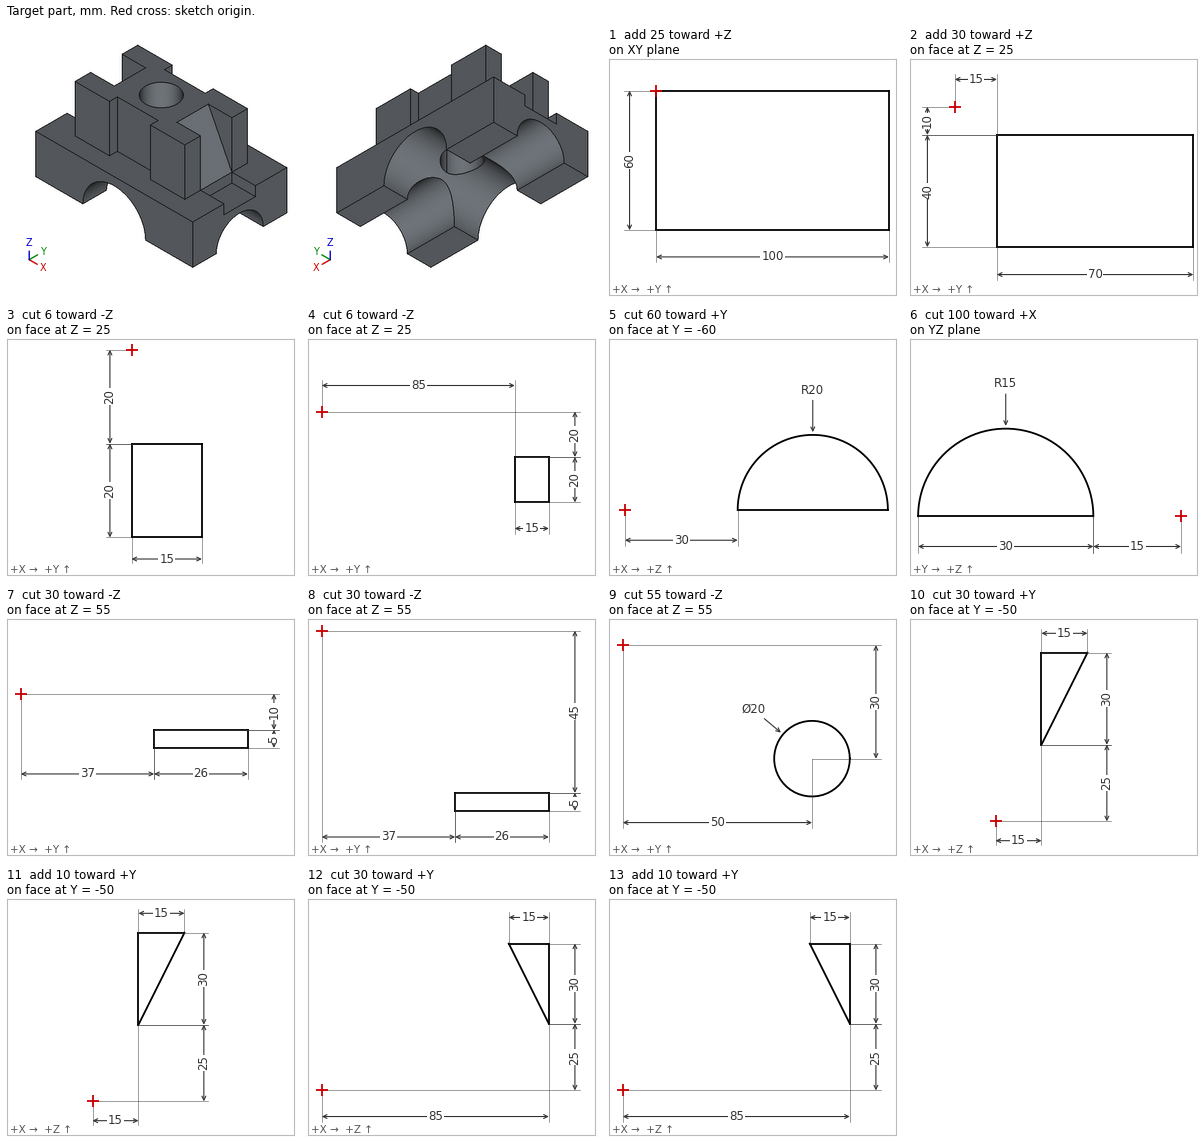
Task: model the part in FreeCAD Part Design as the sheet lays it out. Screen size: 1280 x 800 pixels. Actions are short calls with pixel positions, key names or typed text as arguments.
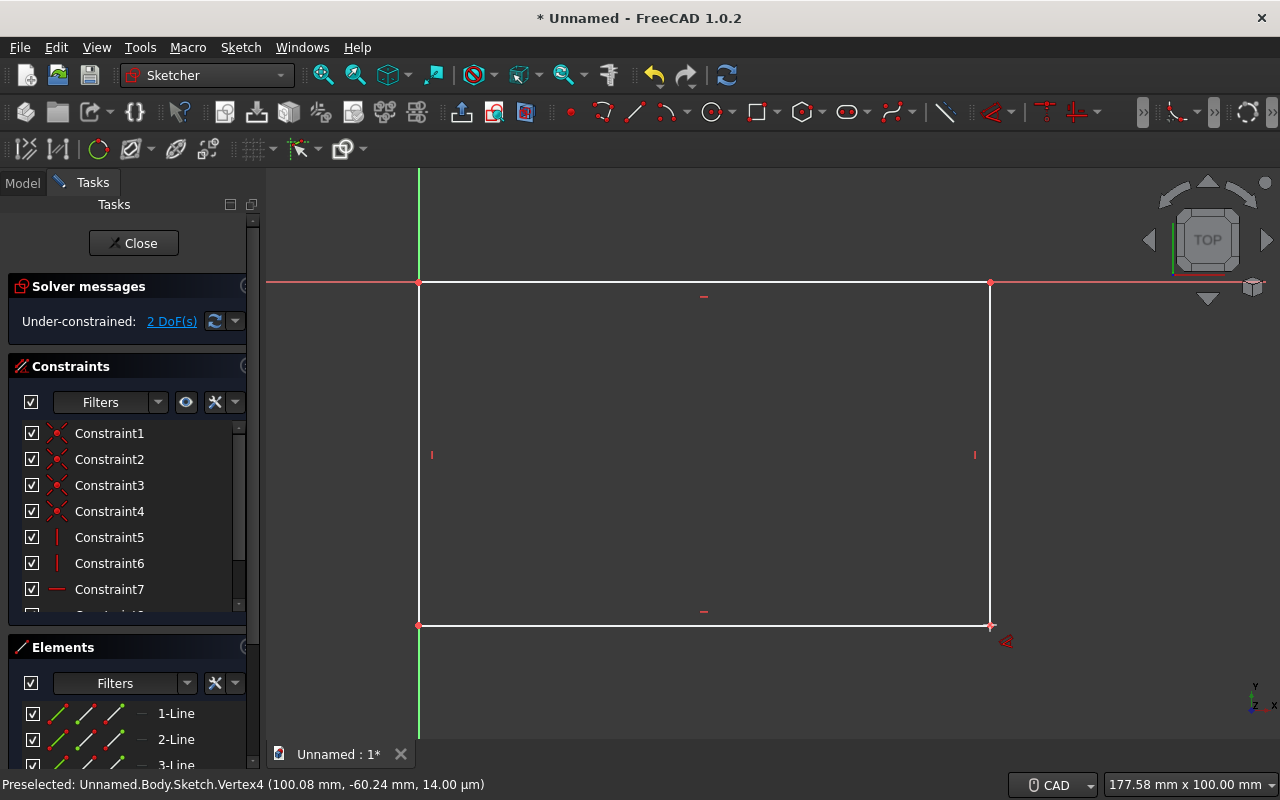
click(419, 385)
click(385, 454)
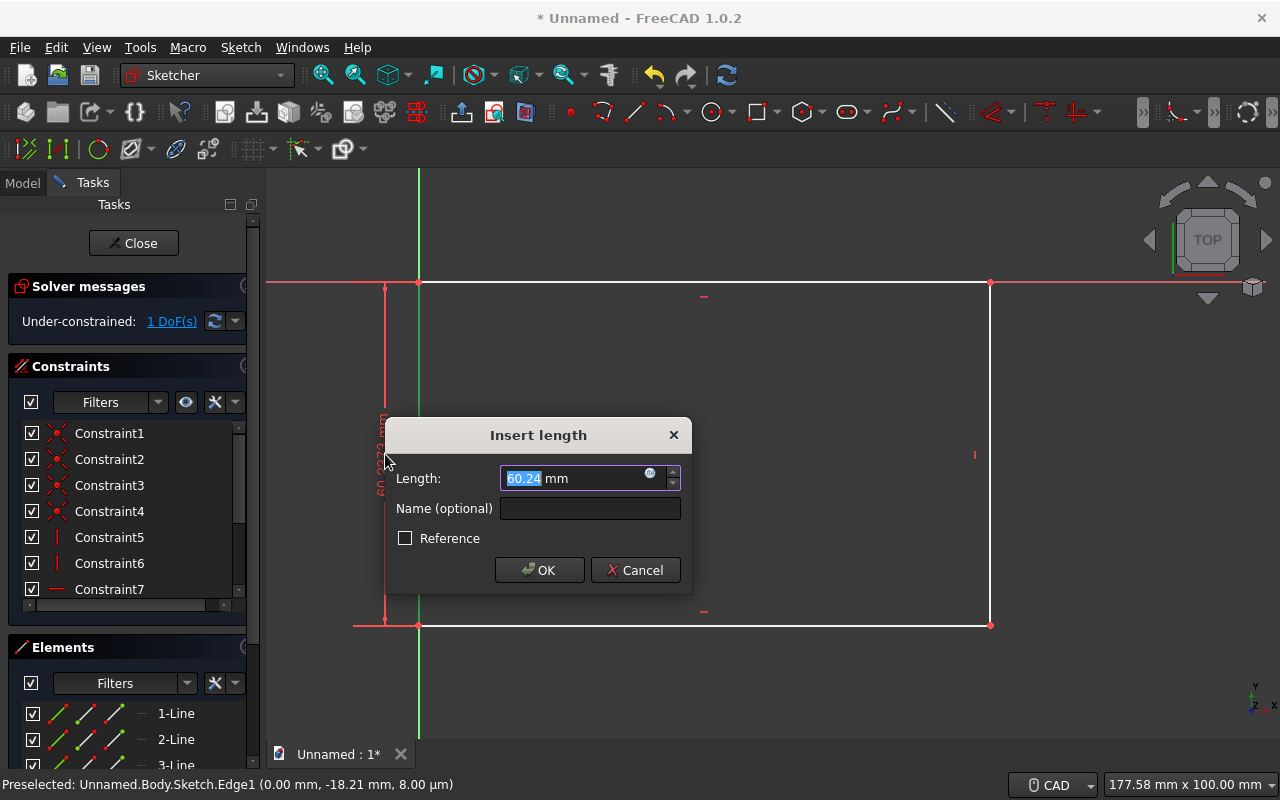
text(60)
key(Return)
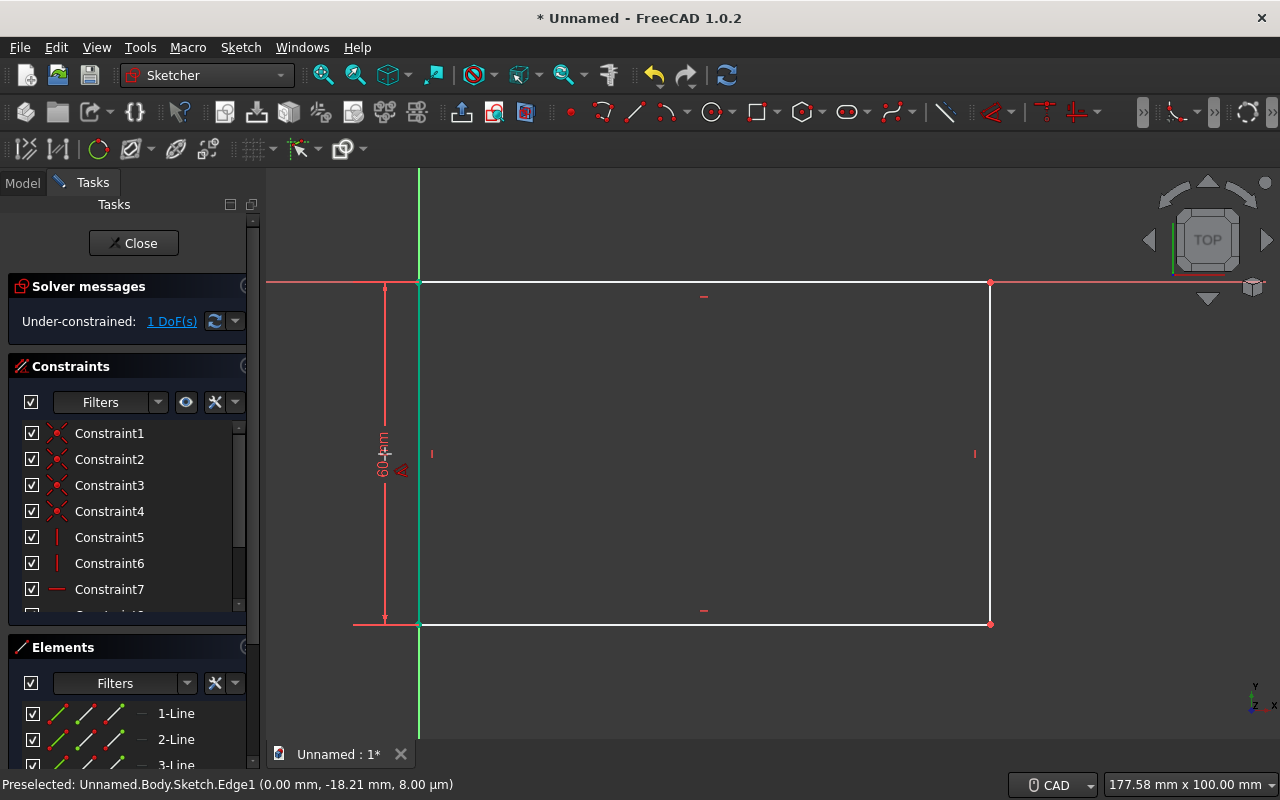
click(590, 625)
click(704, 659)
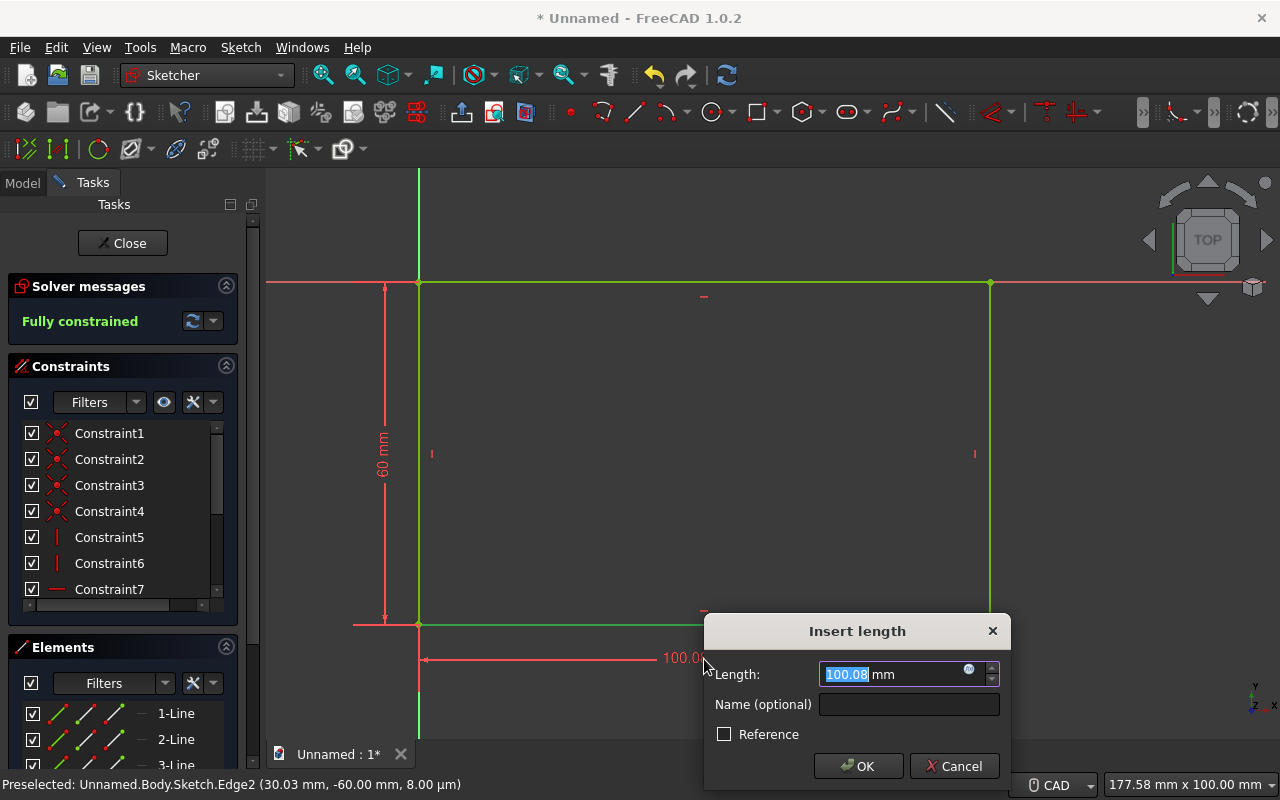
text(100)
key(Return)
key(Escape)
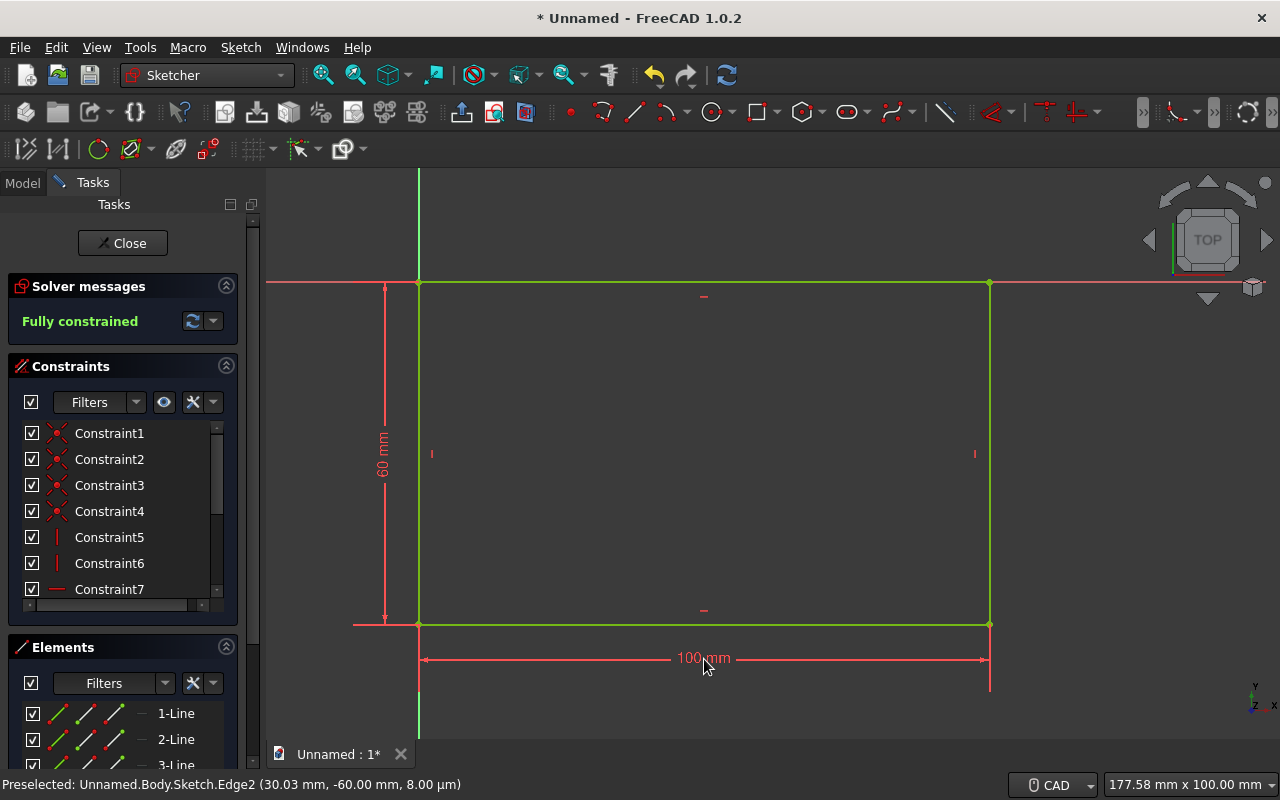
click(123, 243)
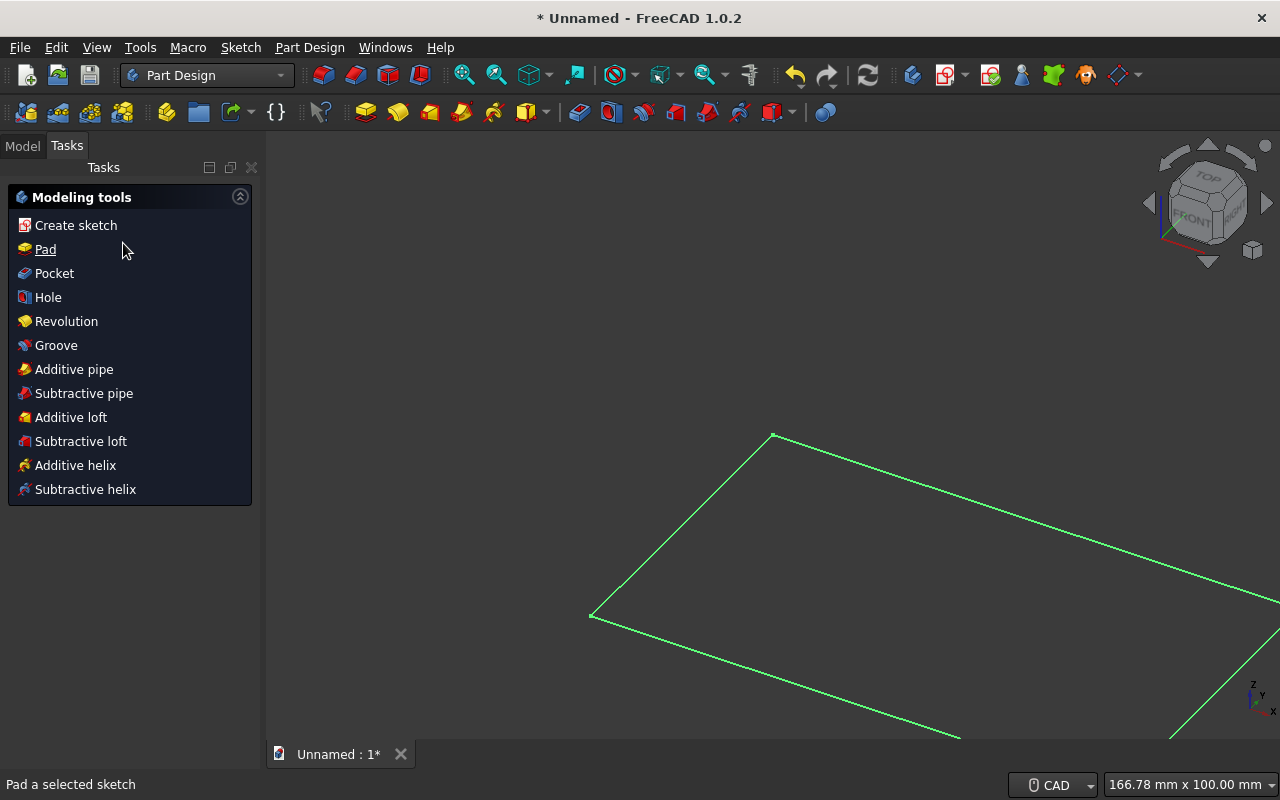
click(366, 112)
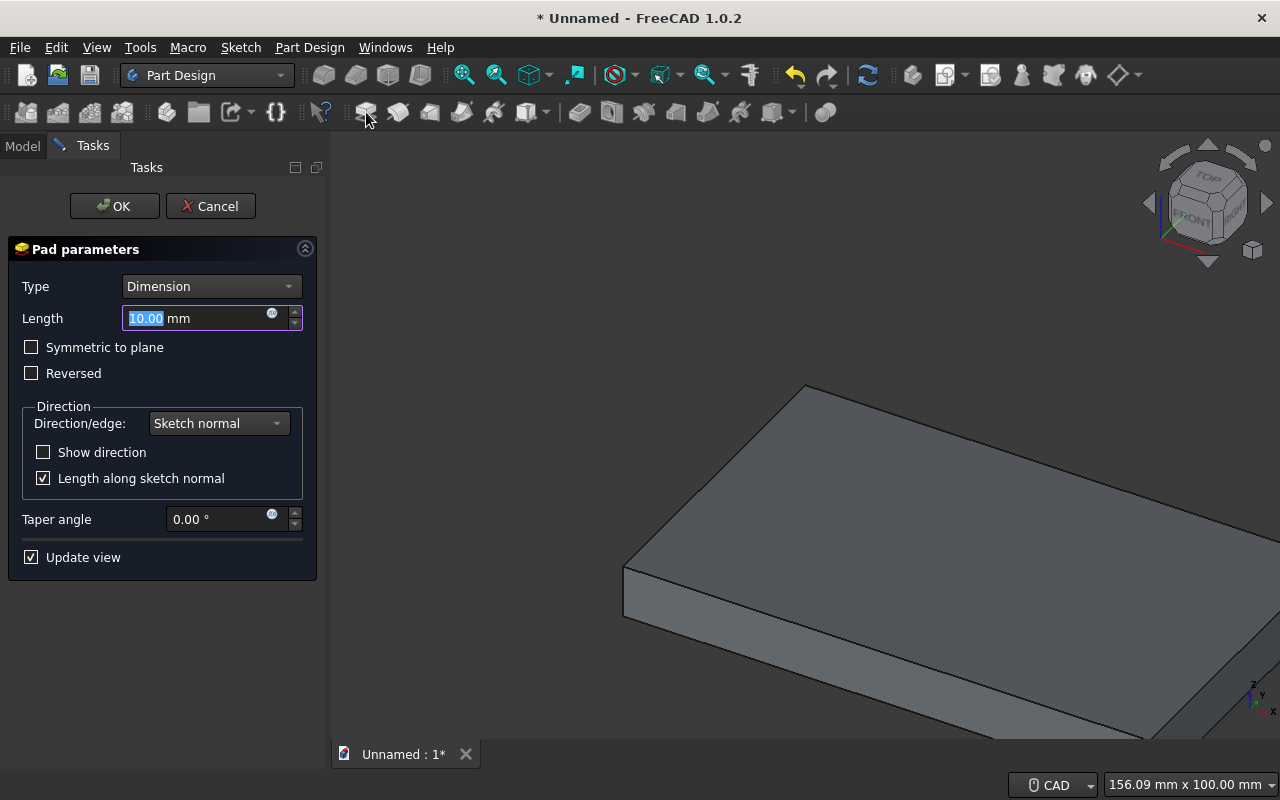
text(25)
key(Tab)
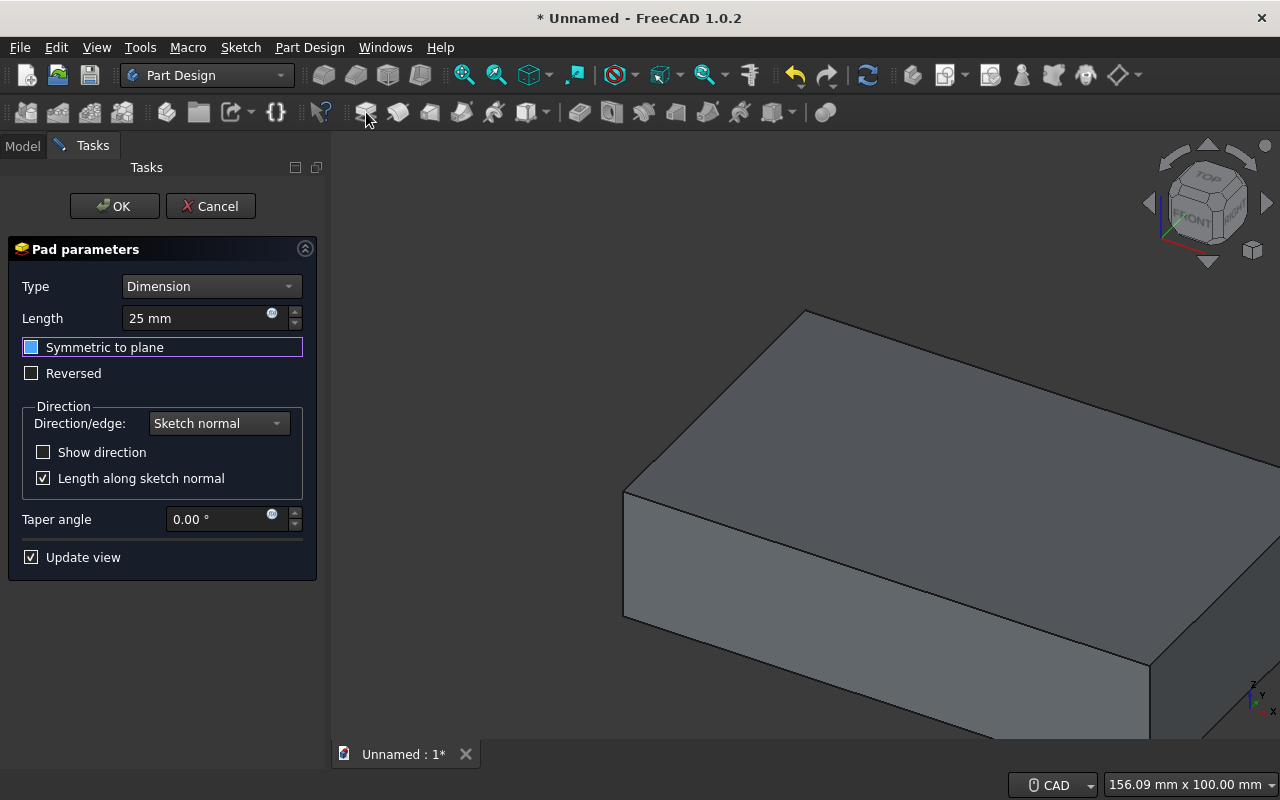
click(115, 206)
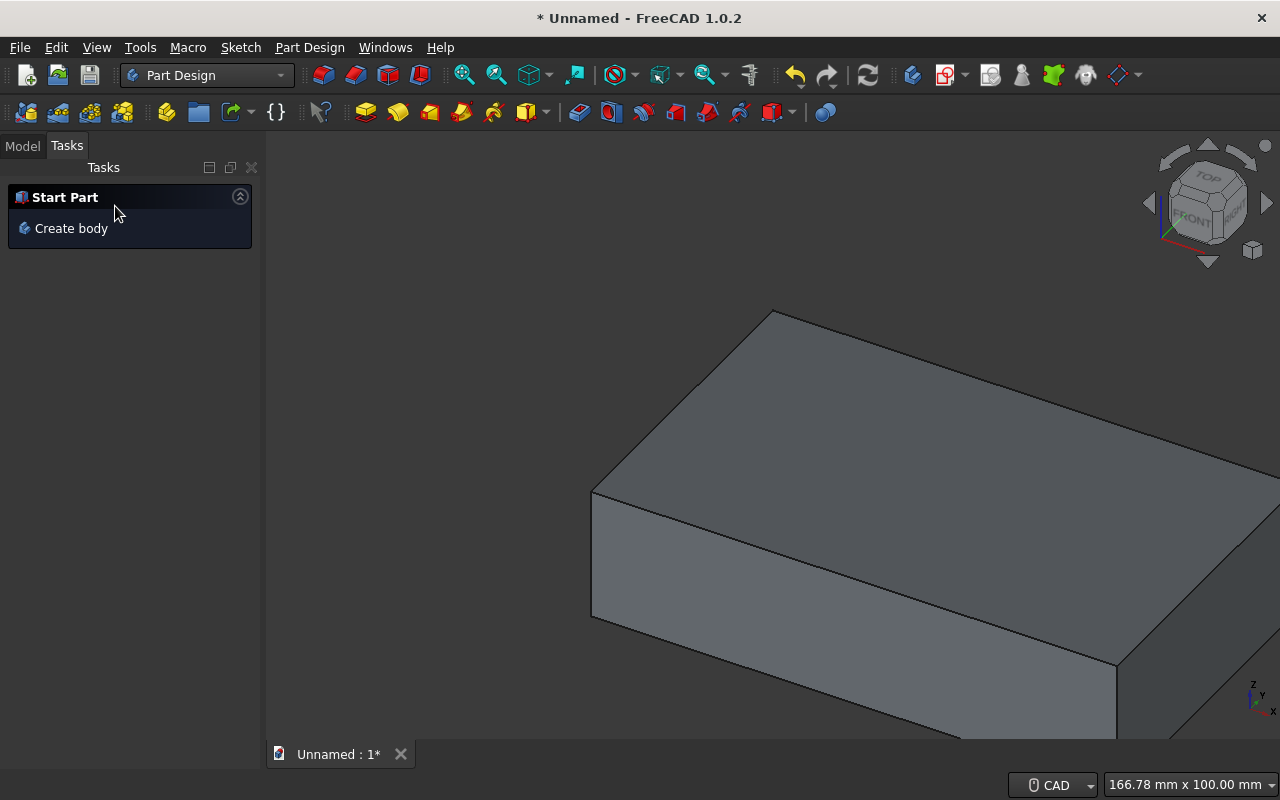
click(466, 76)